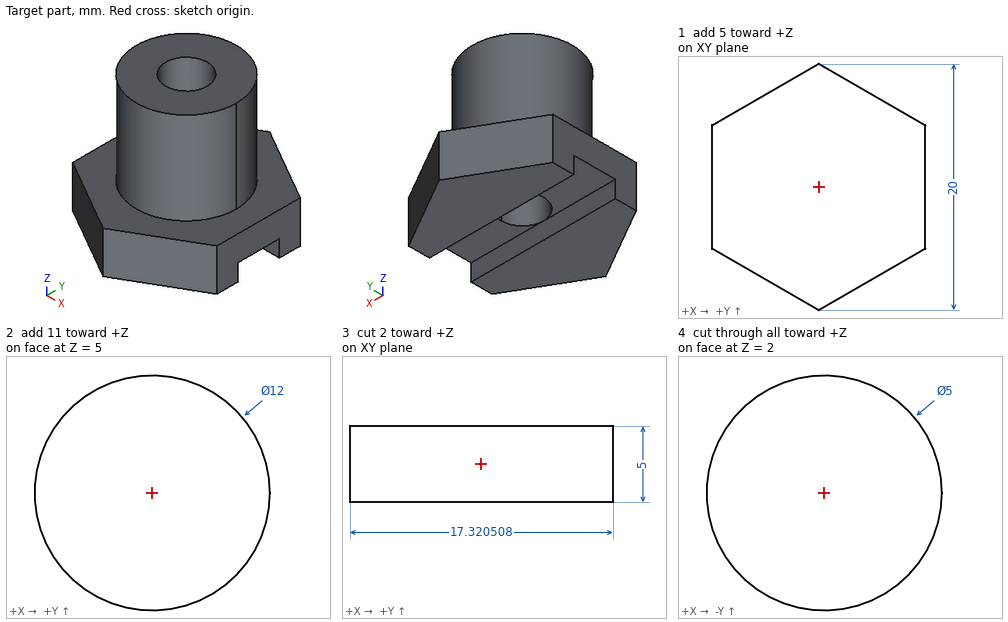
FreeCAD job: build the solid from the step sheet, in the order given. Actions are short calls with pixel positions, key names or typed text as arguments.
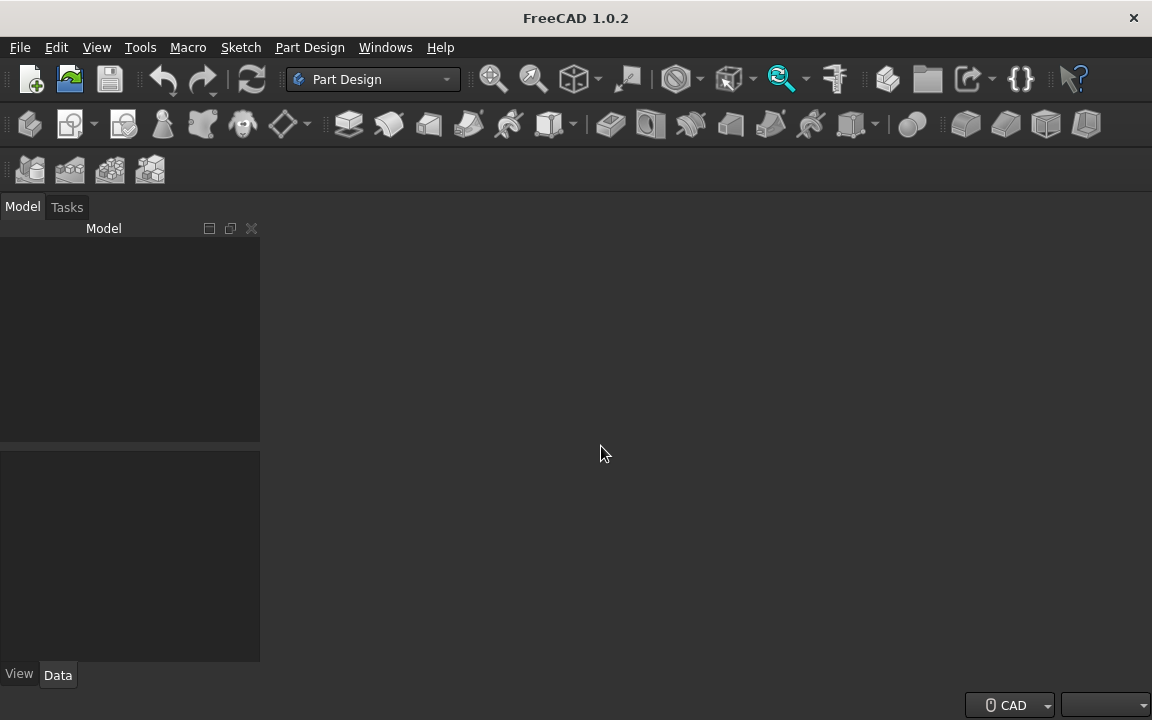
key(ctrl+n)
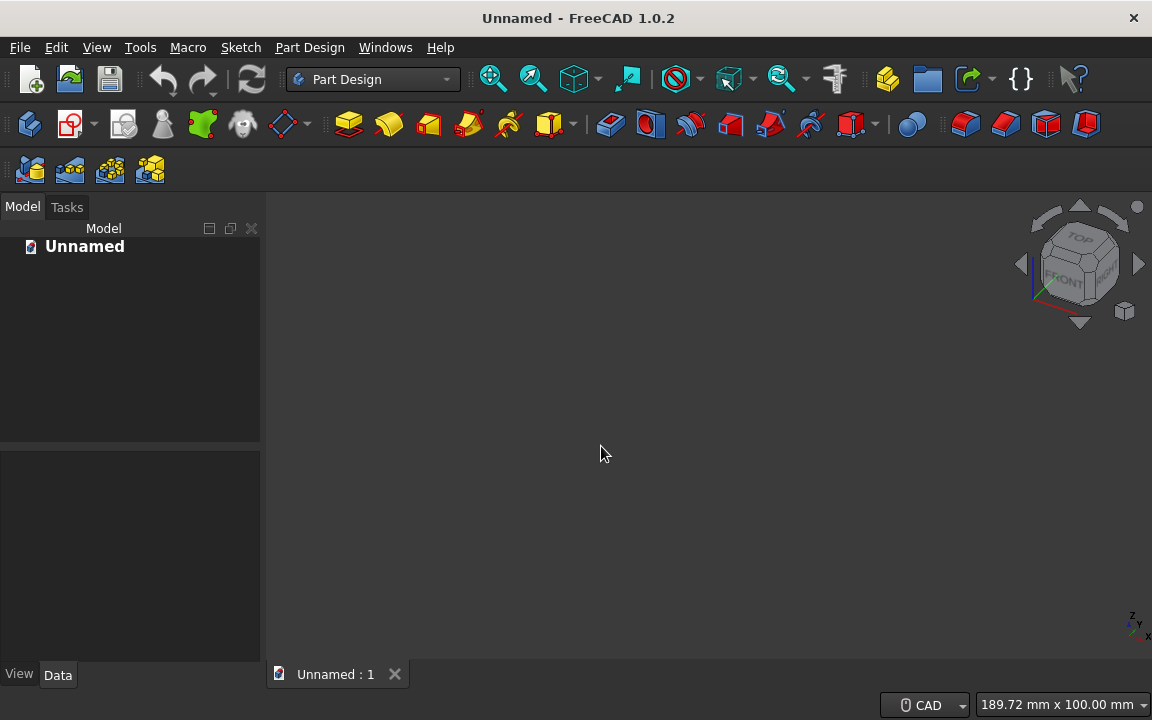
click(70, 124)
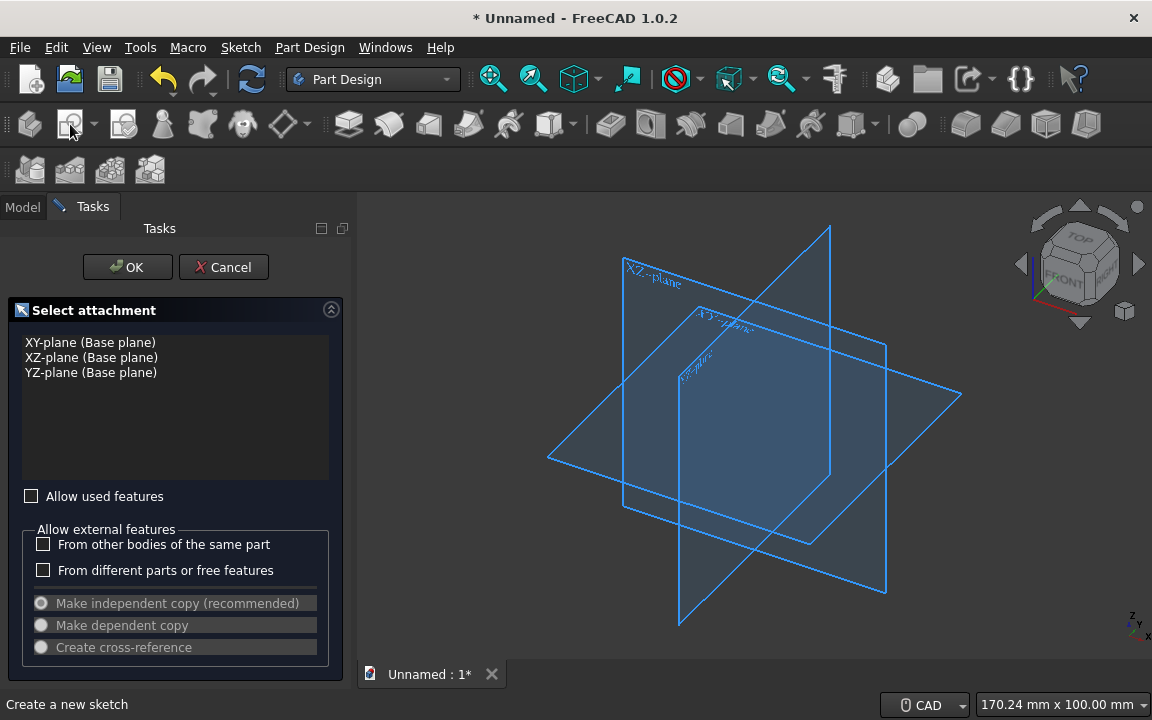
click(82, 342)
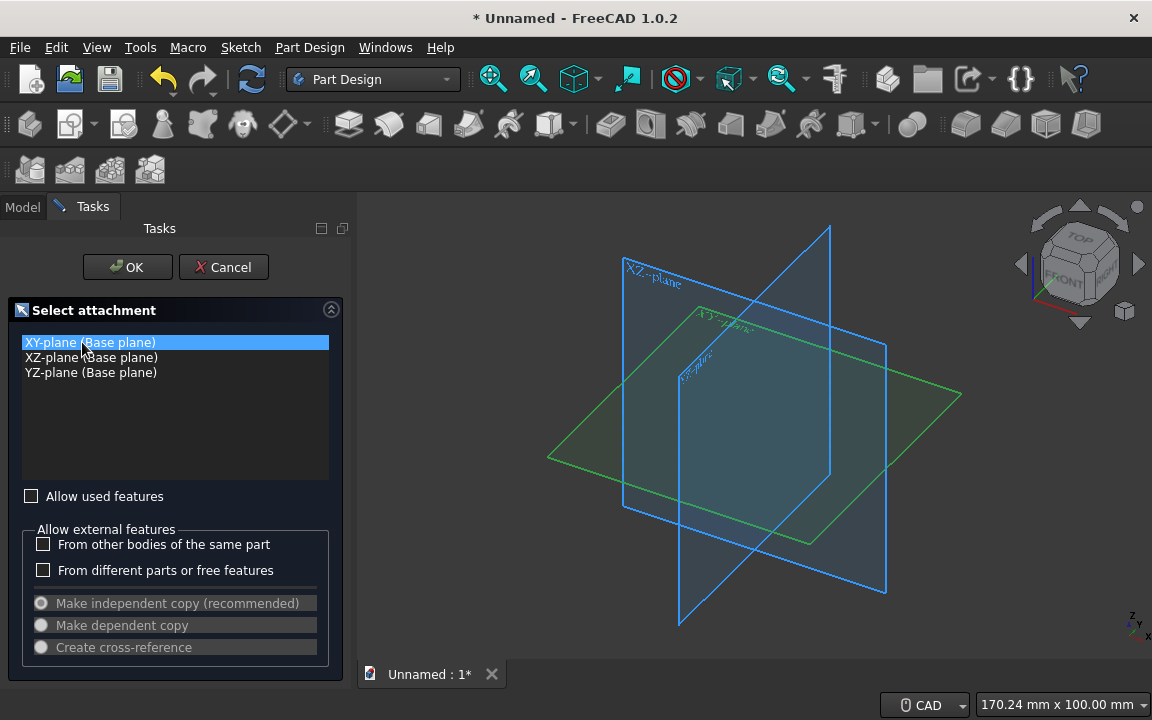
click(128, 267)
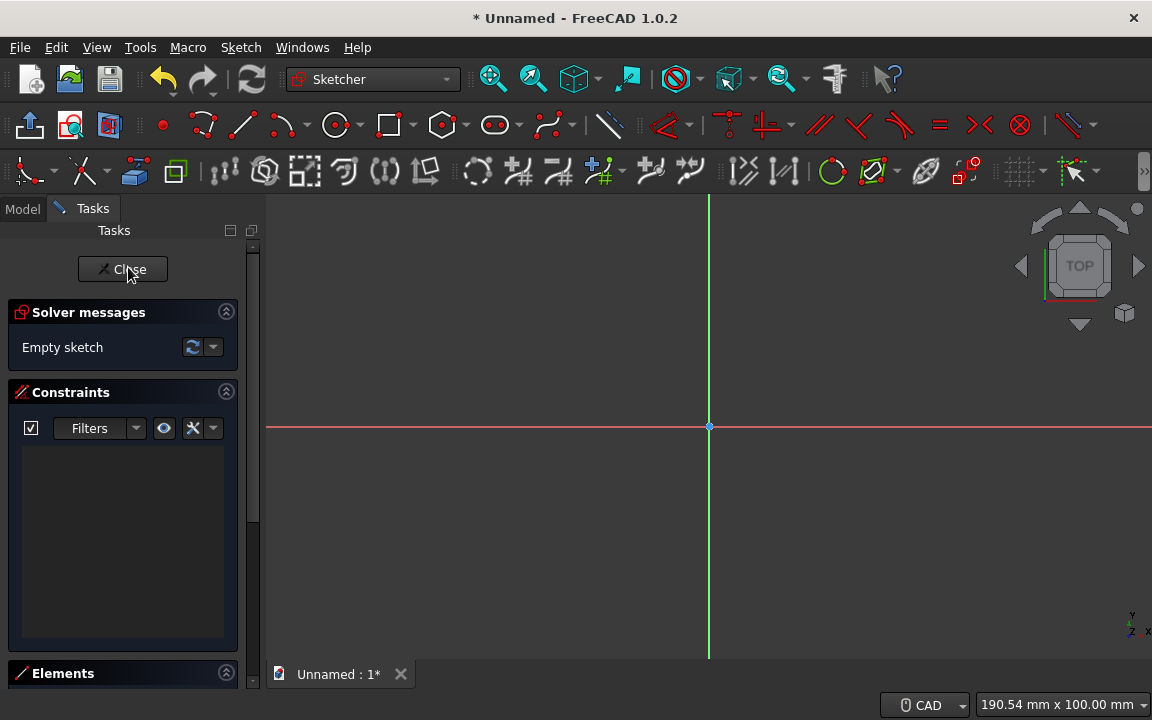
scroll(739, 427, up, 6)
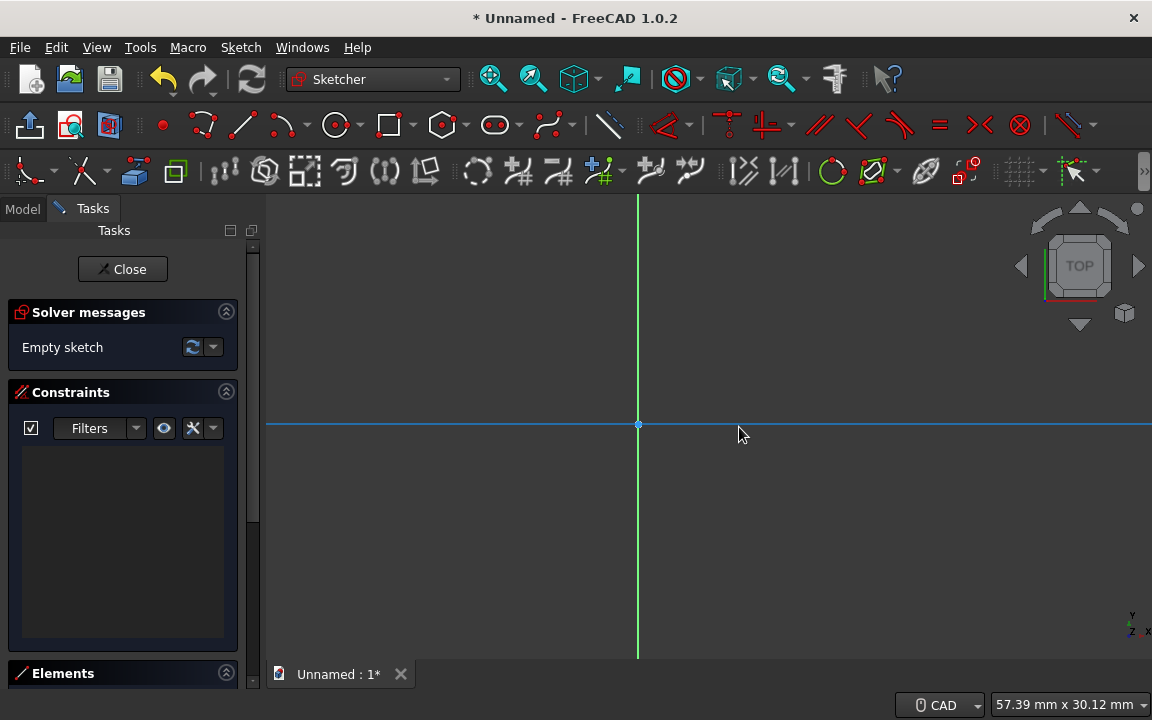
key(g)
key(p)
key(6)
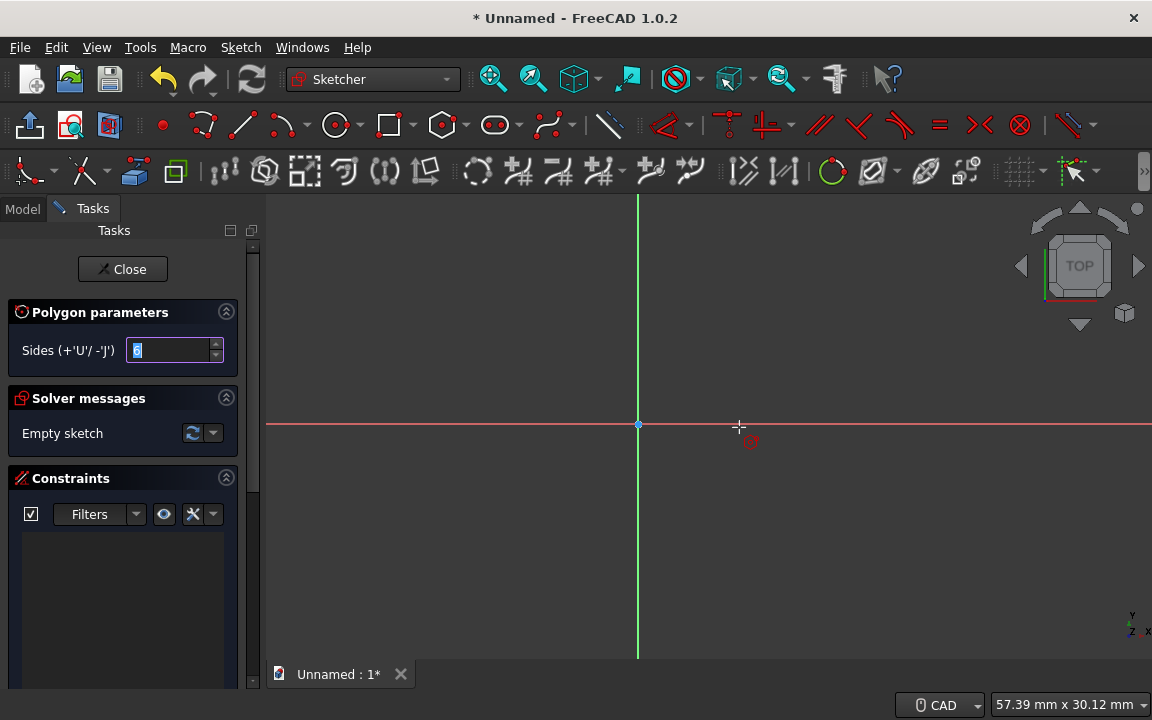
click(638, 424)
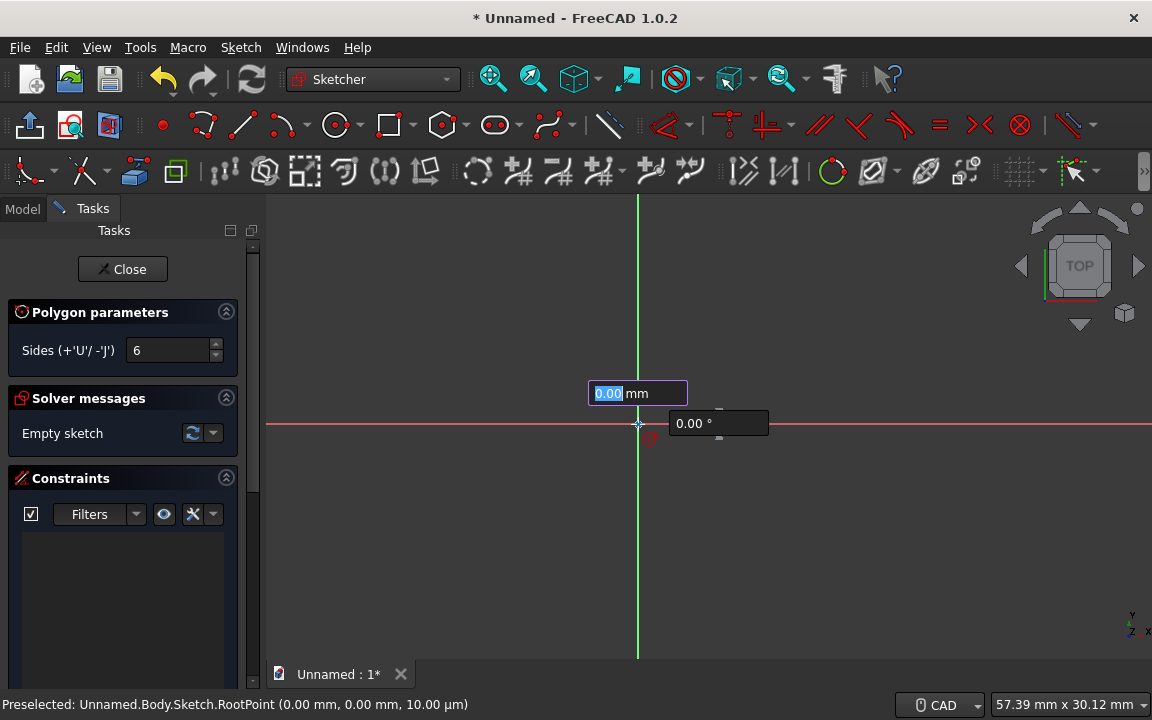
click(638, 270)
right_click(638, 270)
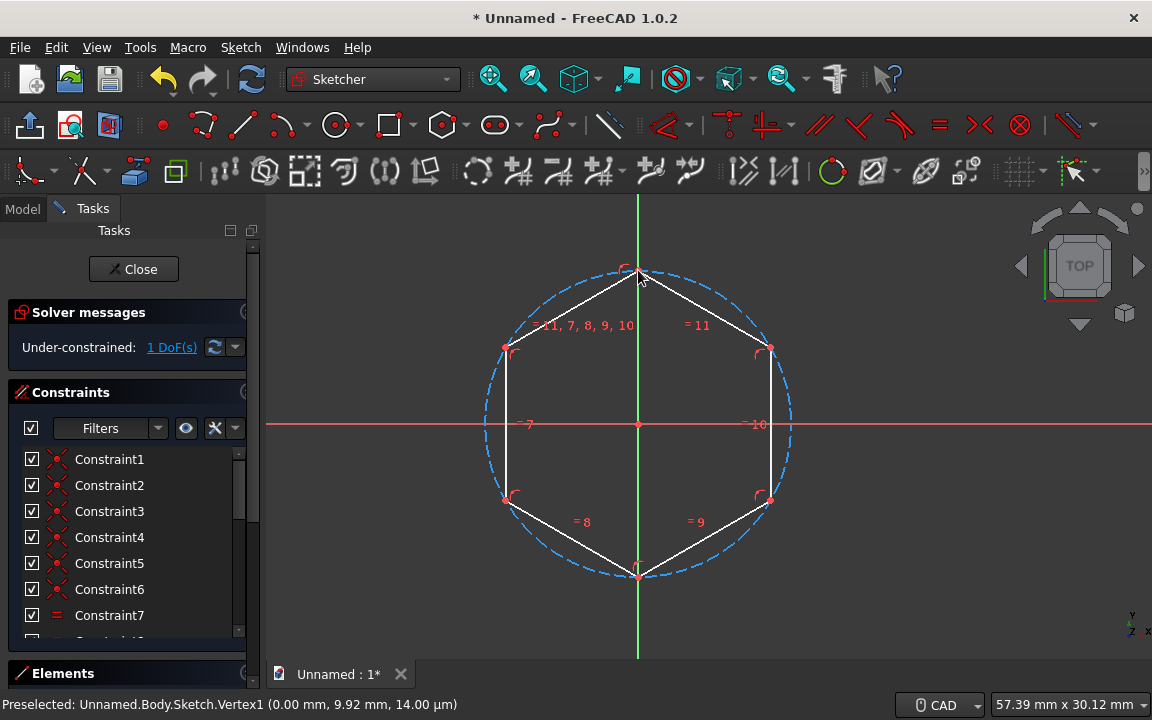
key(d)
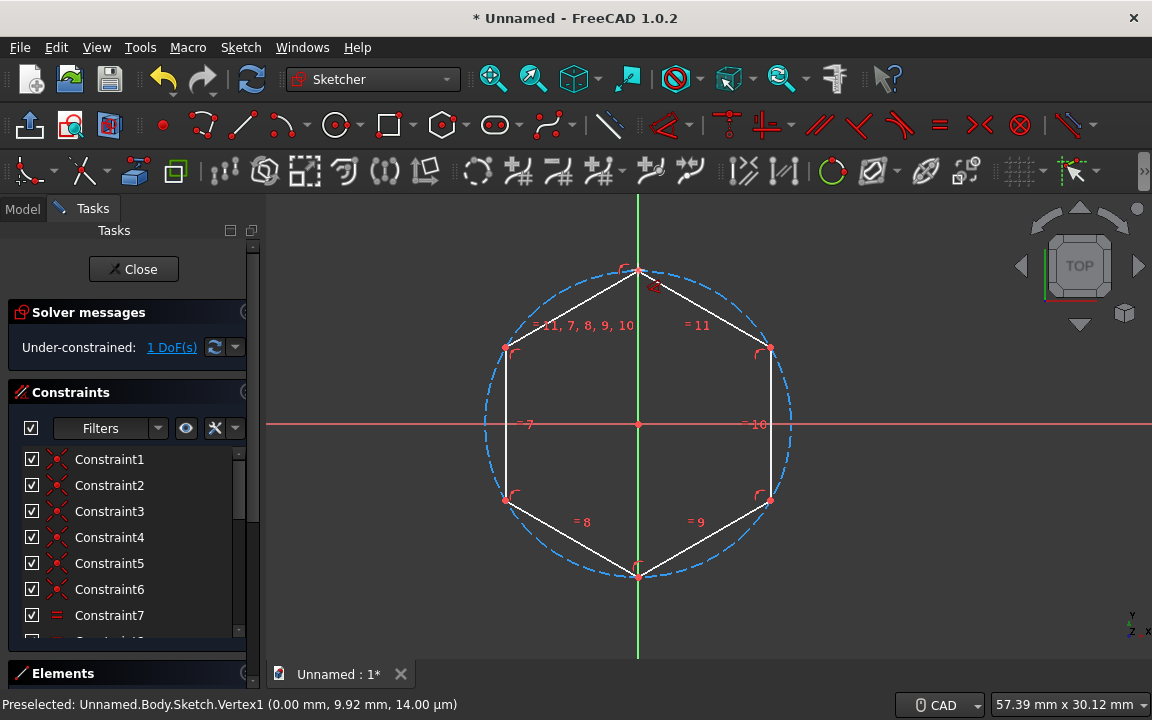
click(638, 577)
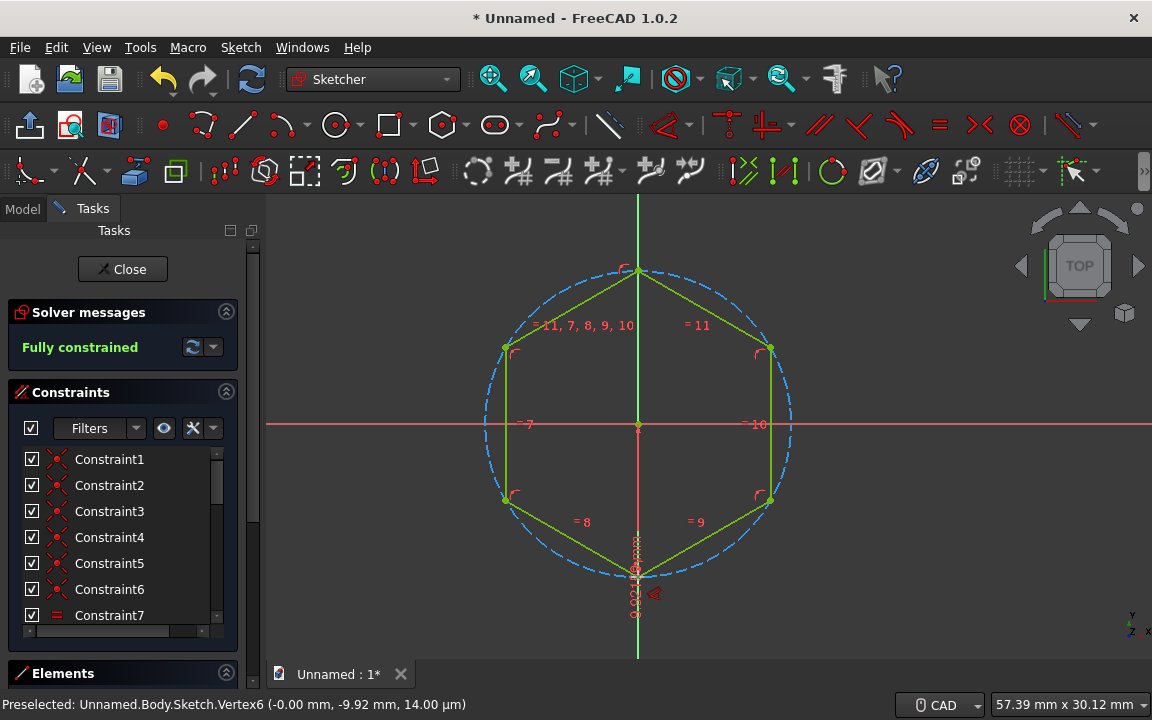
click(638, 271)
click(672, 354)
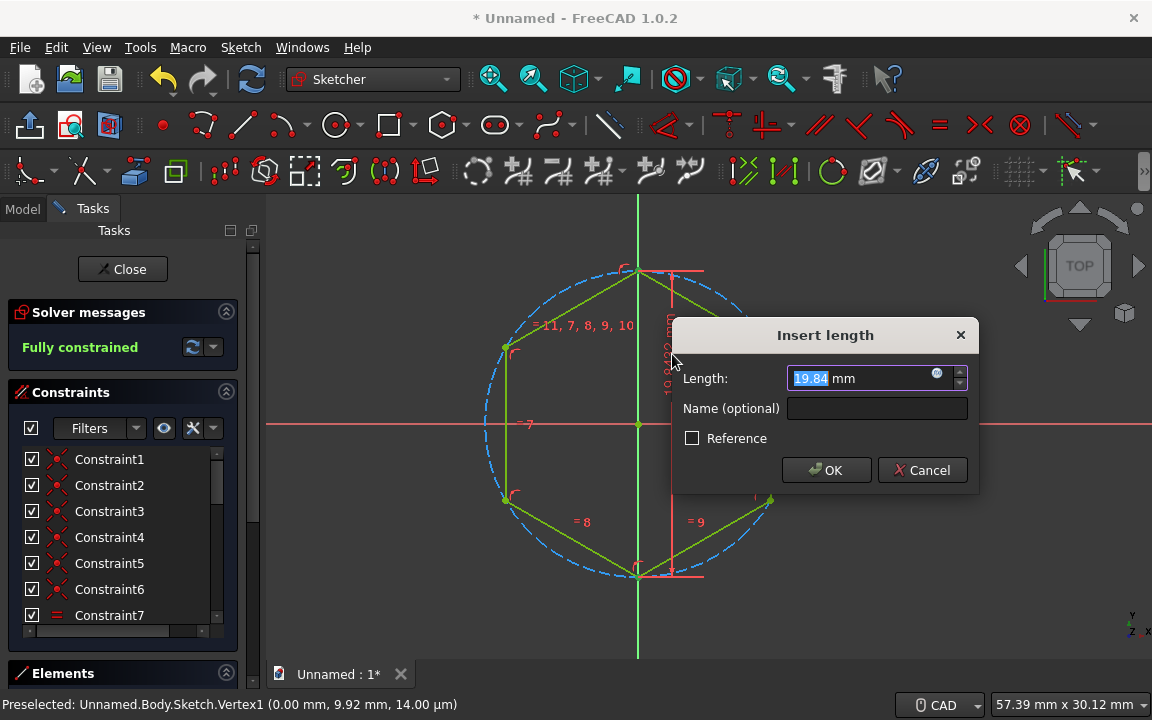
text(20)
key(Return)
key(Escape)